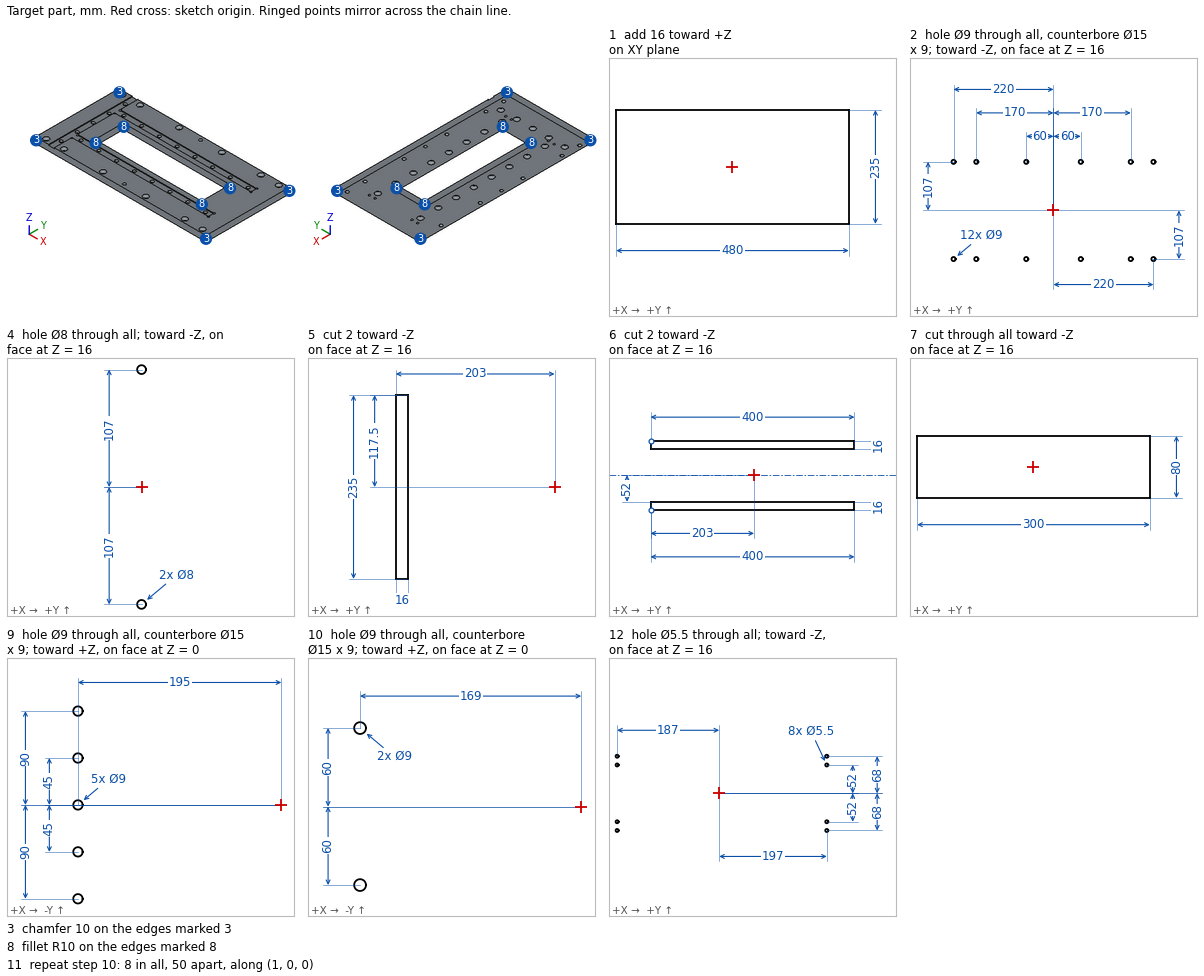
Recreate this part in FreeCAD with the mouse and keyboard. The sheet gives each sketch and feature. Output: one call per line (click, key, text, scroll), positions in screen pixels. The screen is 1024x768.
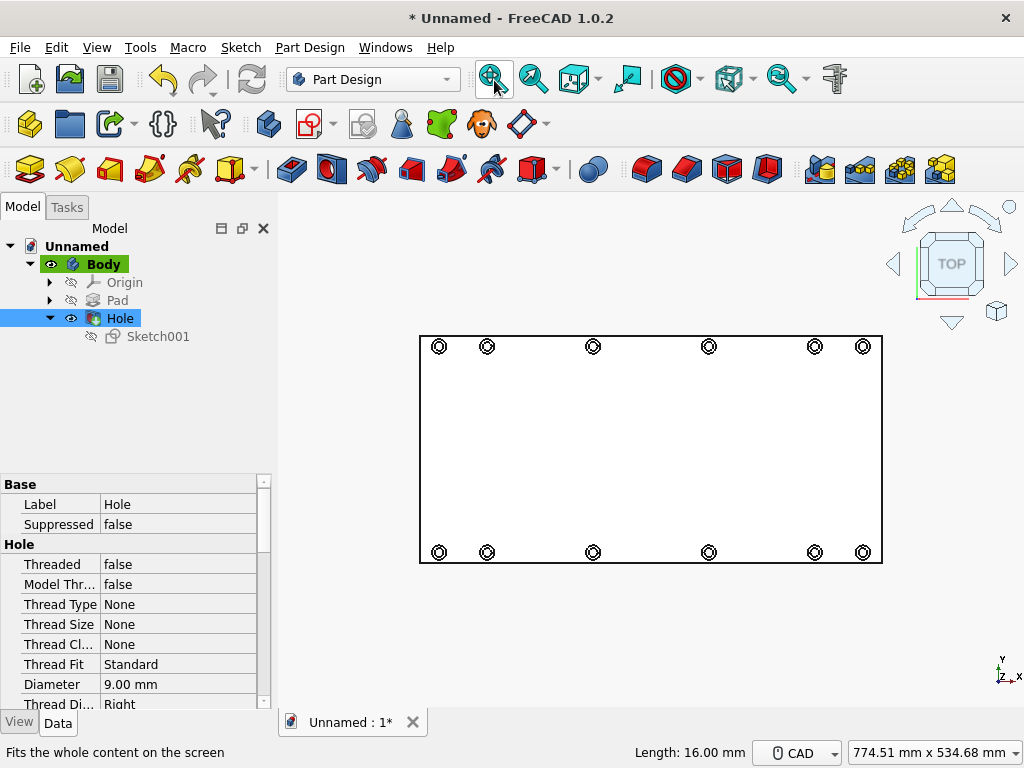
scroll(420, 335, up, 5)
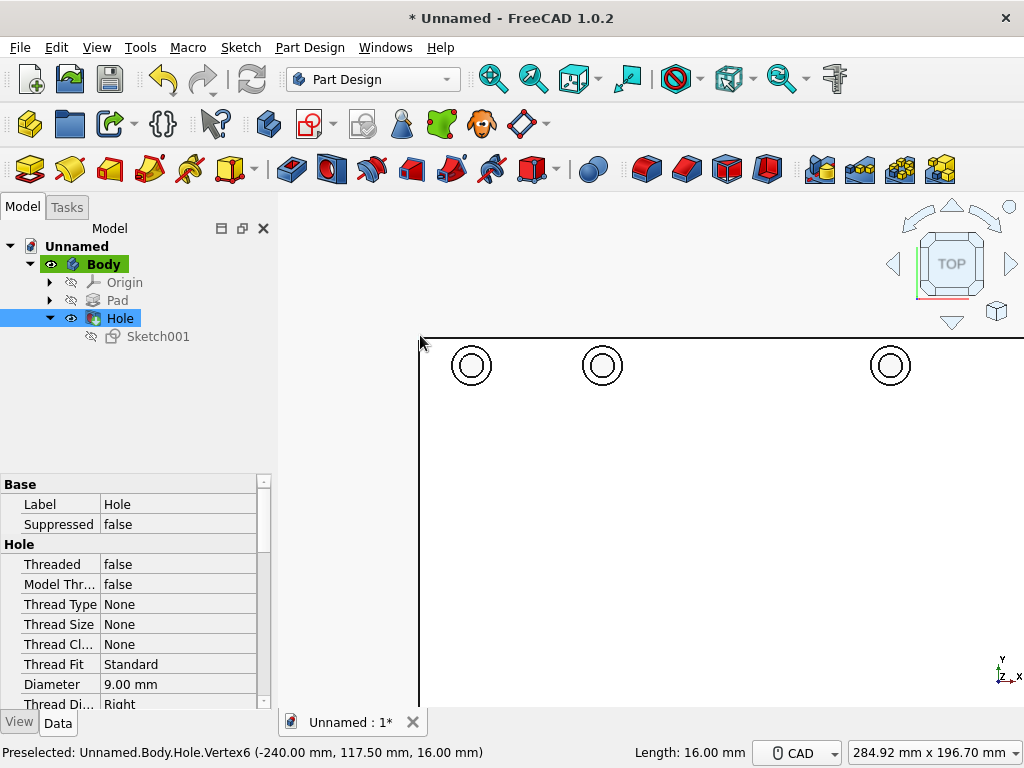
click(494, 80)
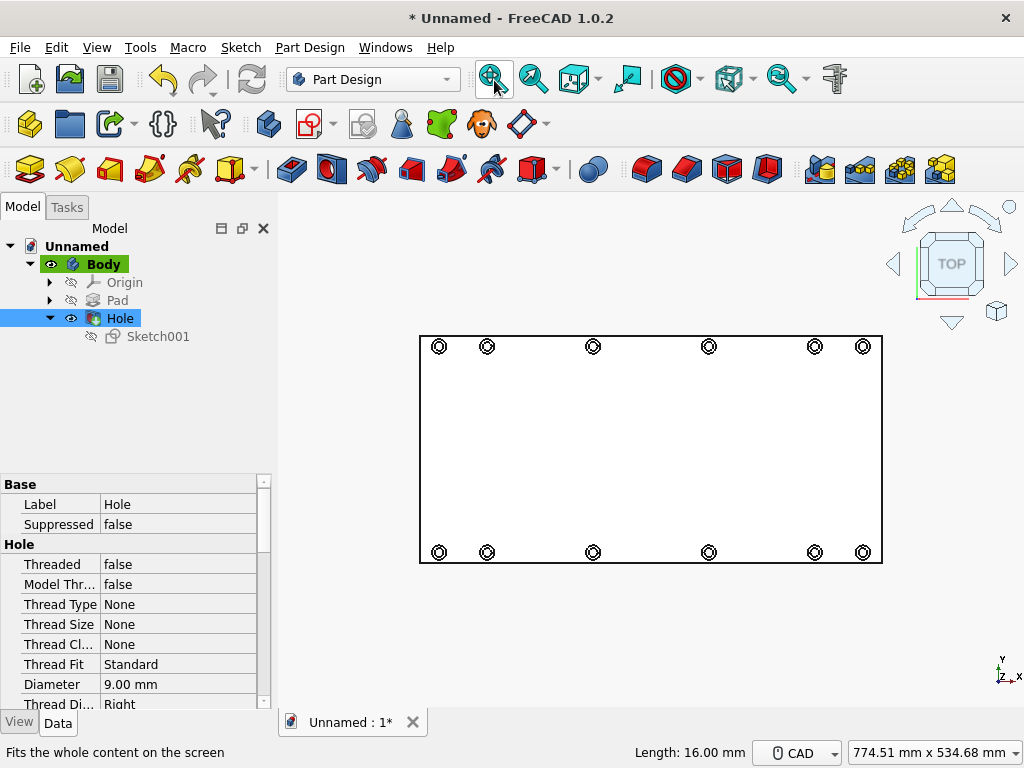
key(1)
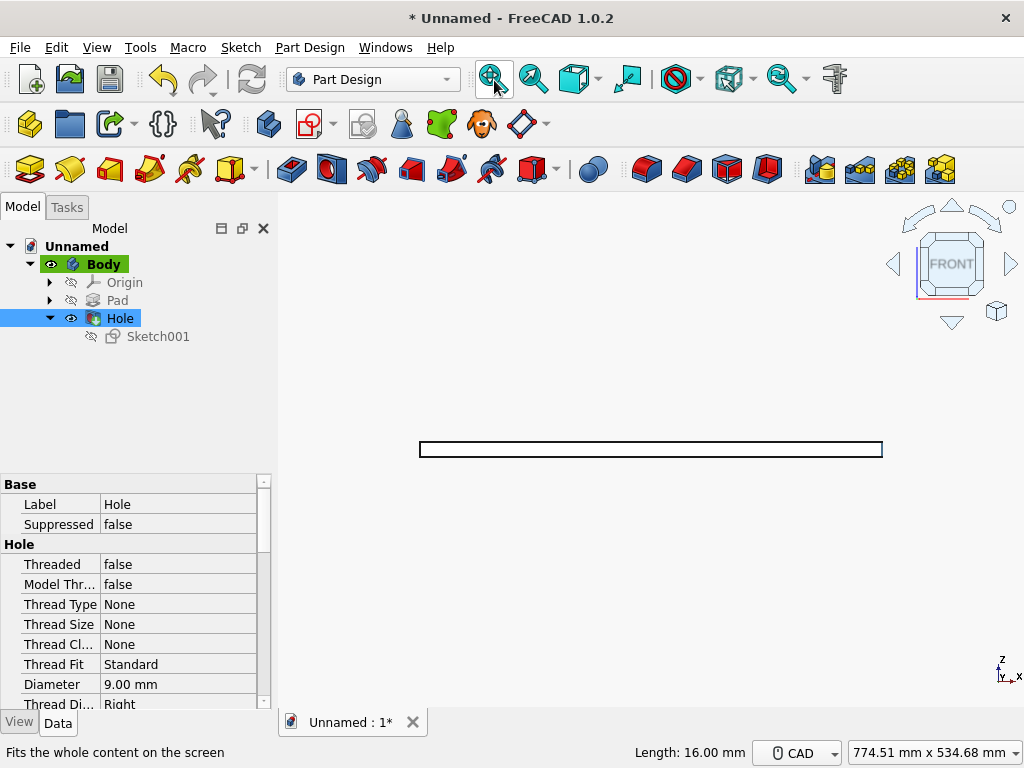
click(420, 449, ctrl)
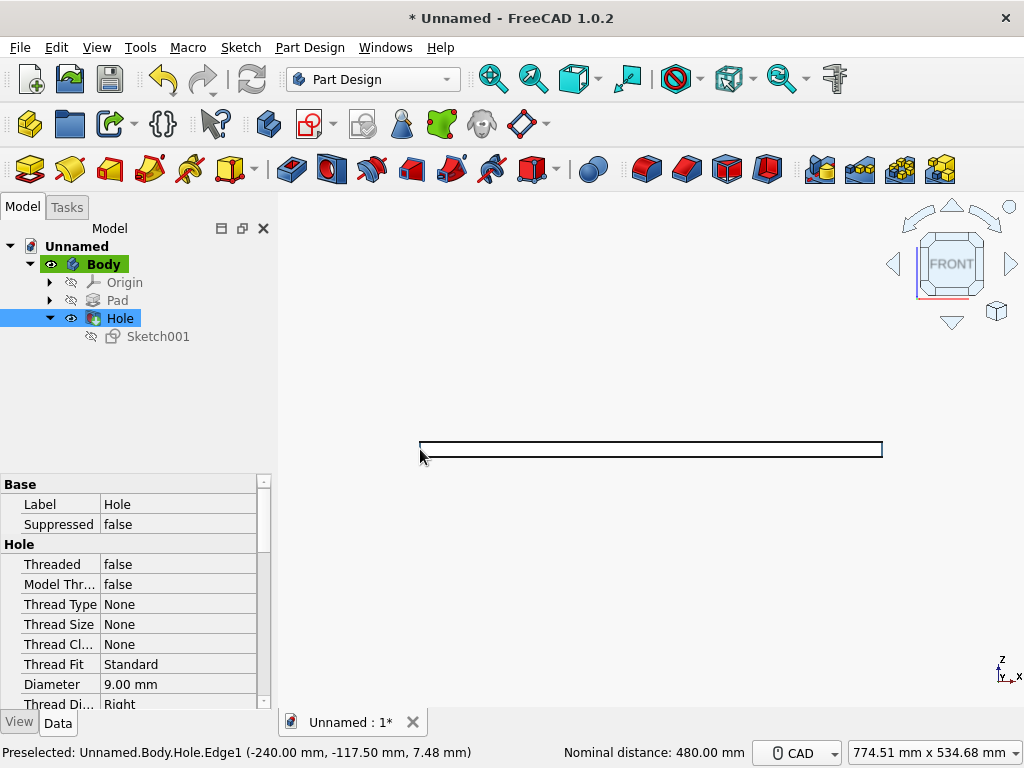
scroll(420, 449, up, 5)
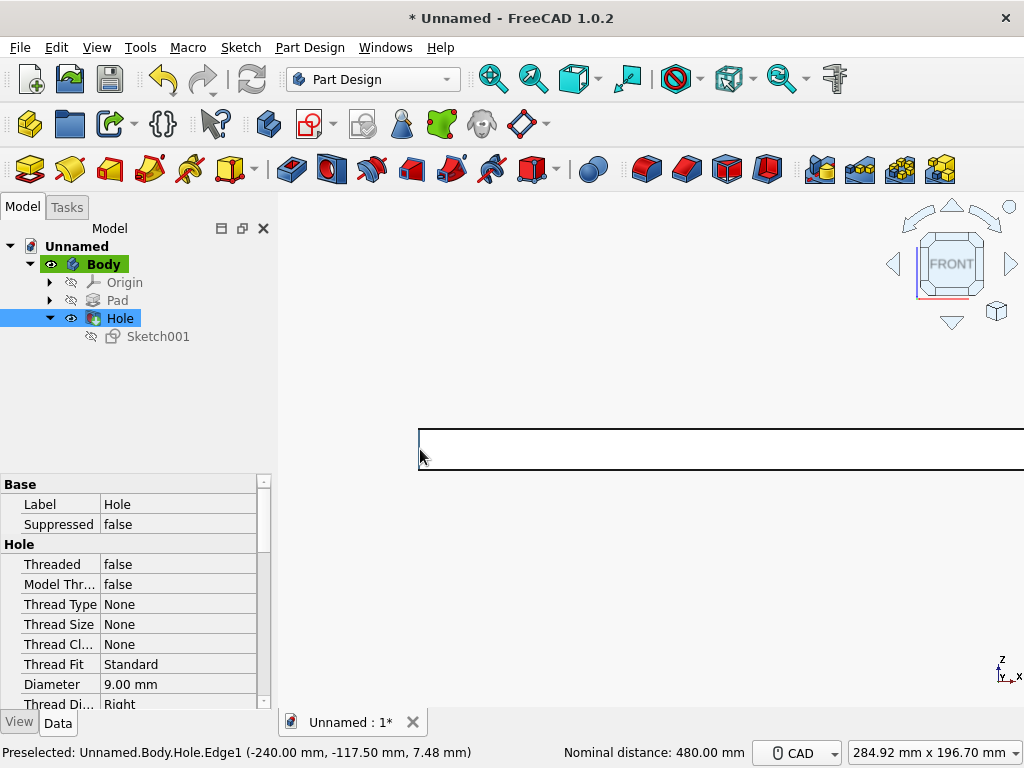
click(494, 80)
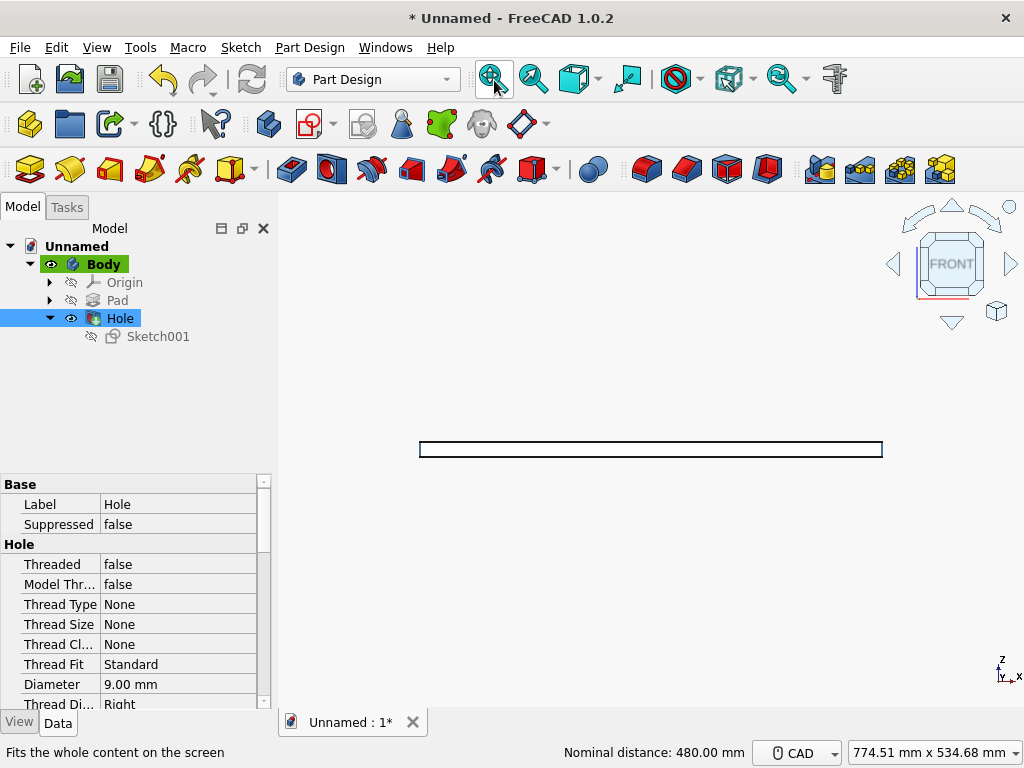
key(3)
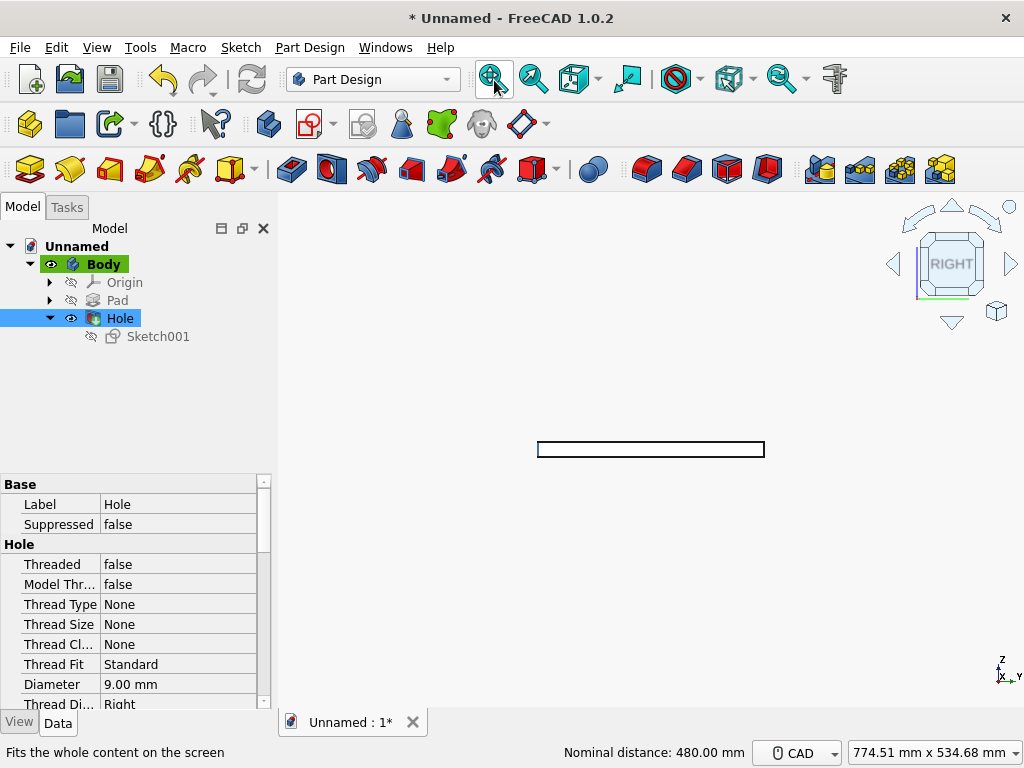
click(494, 80)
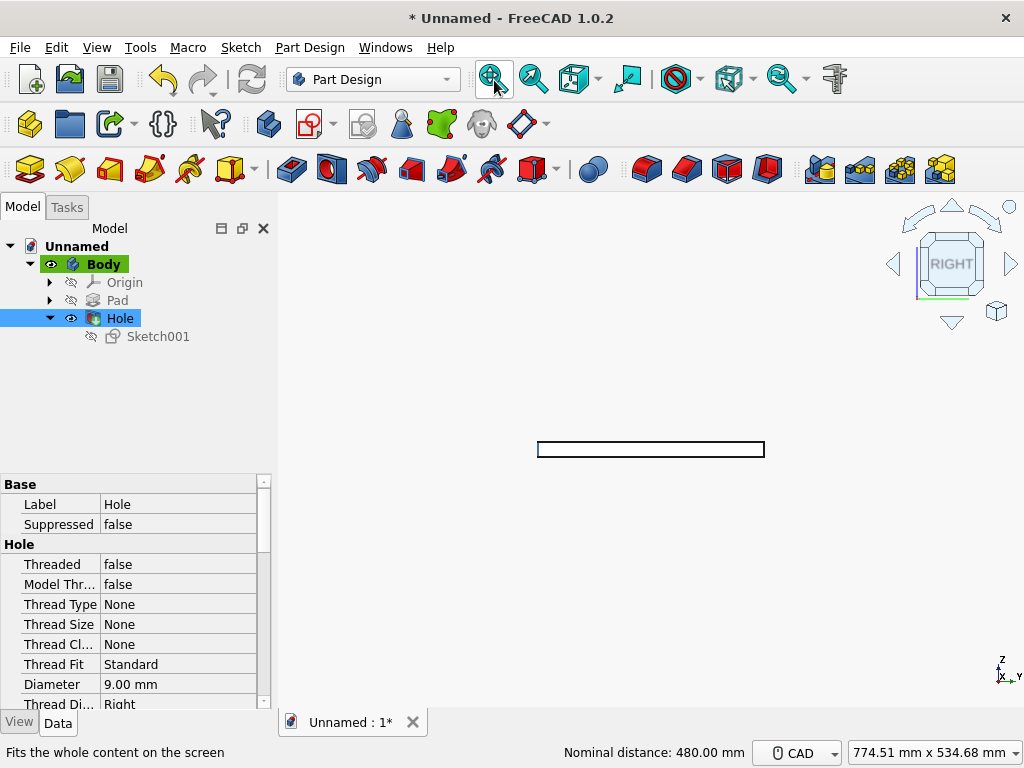
click(764, 448, ctrl)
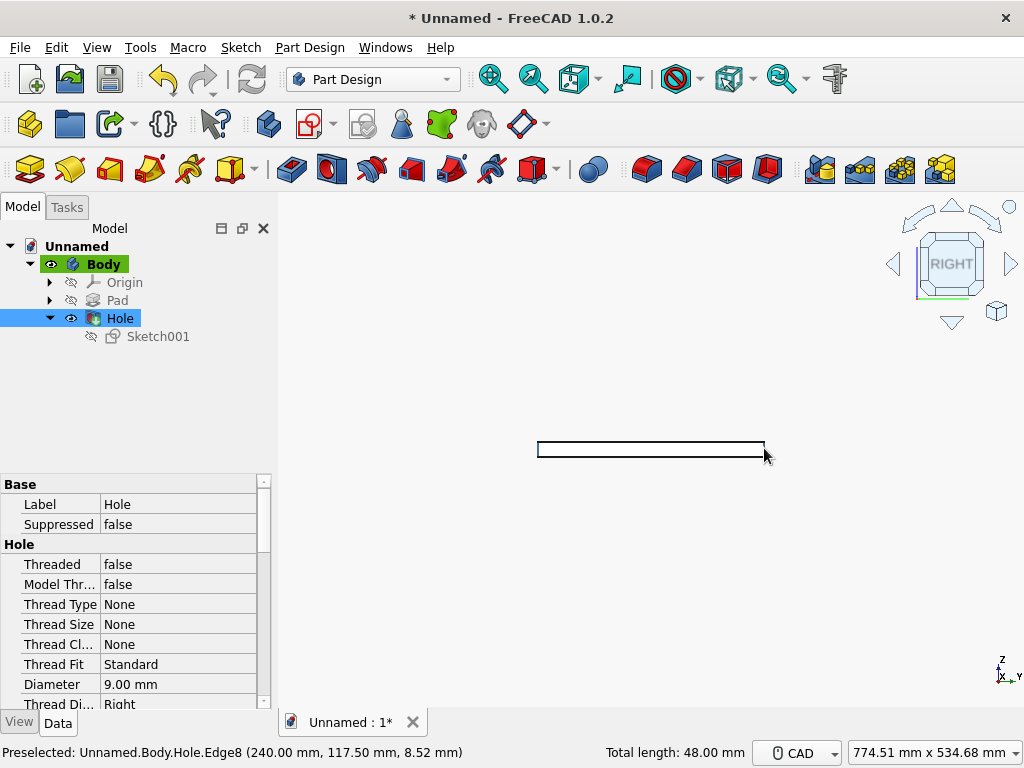
scroll(764, 448, up, 5)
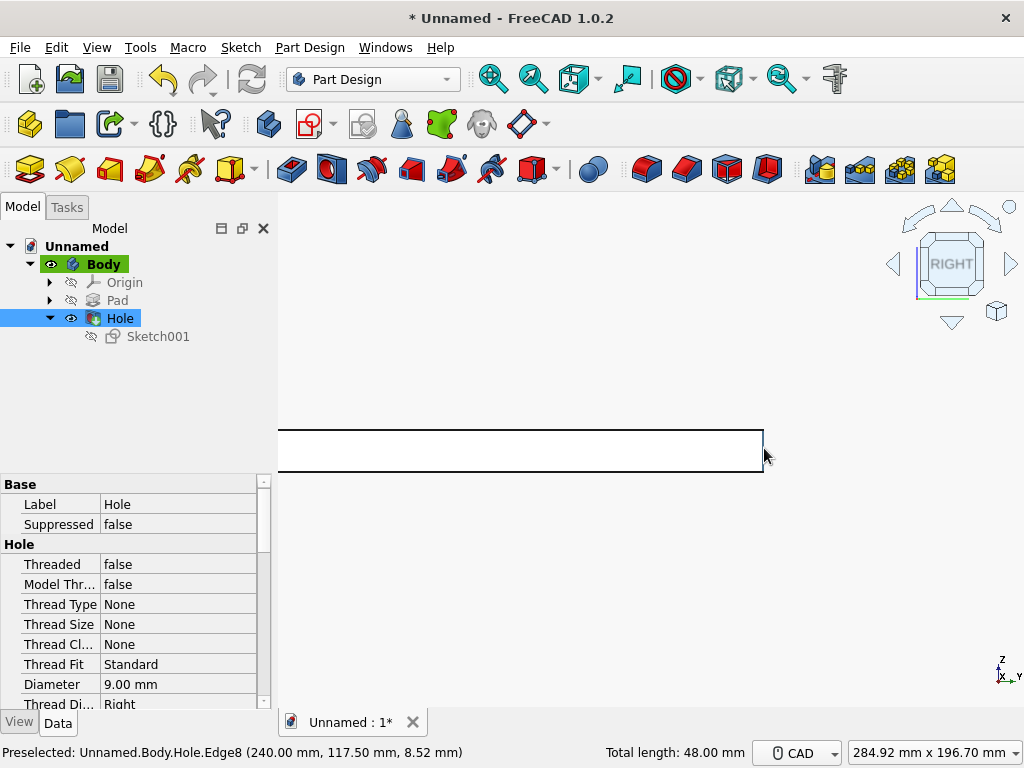
click(494, 80)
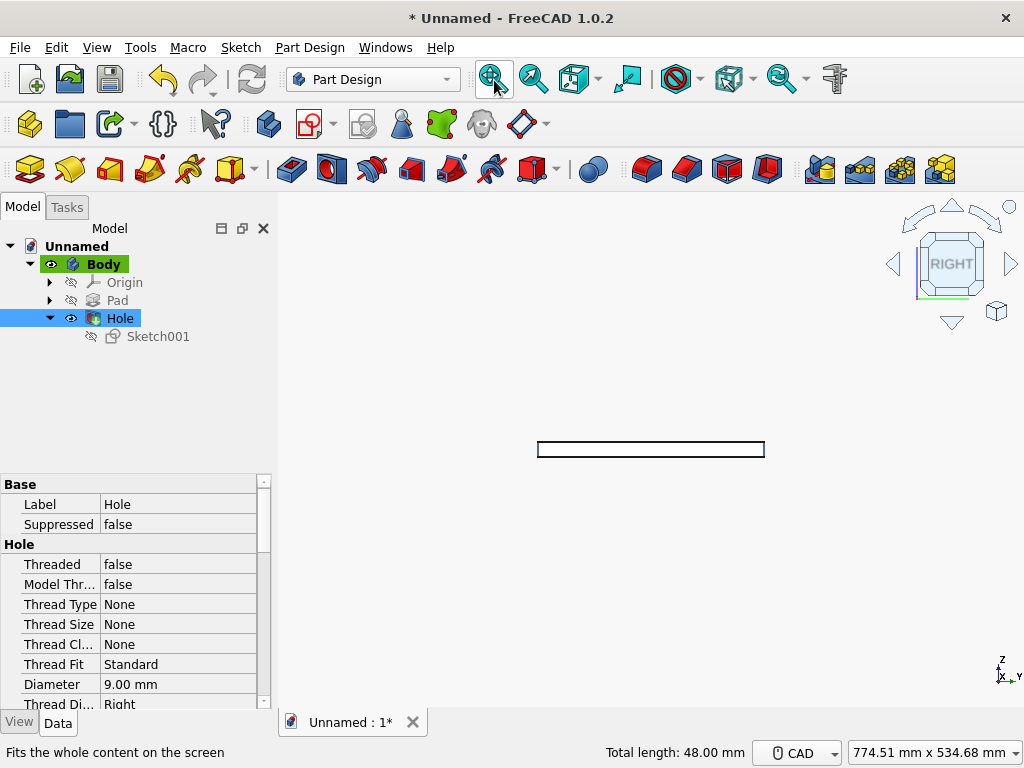
key(5)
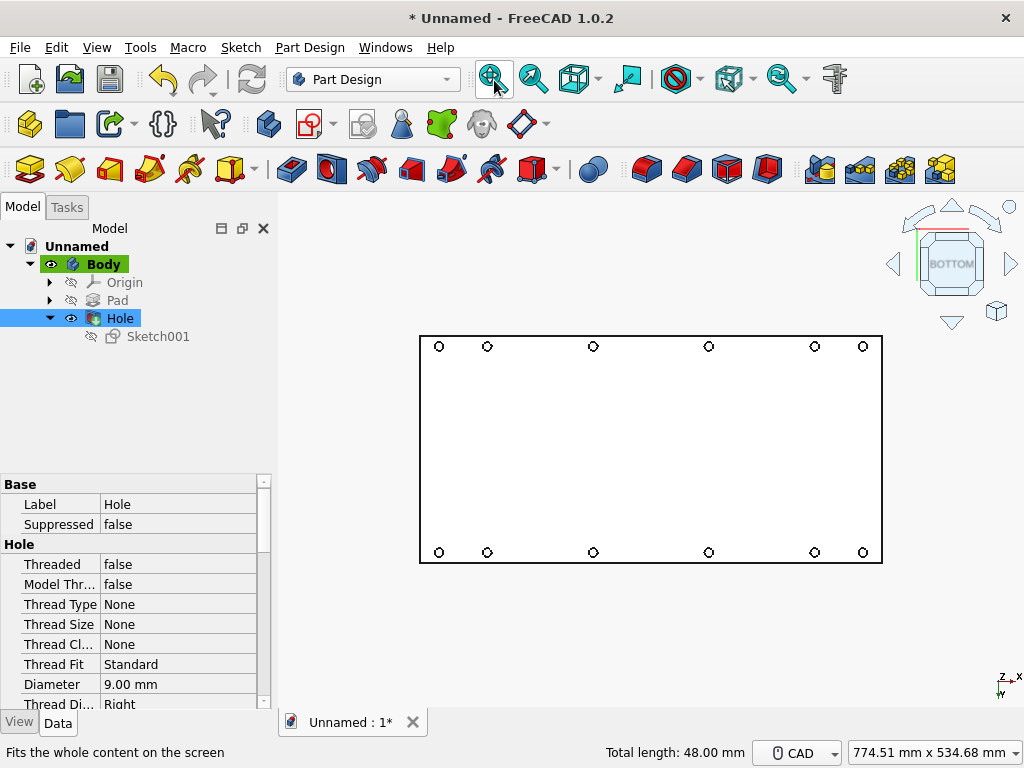
scroll(420, 562, up, 5)